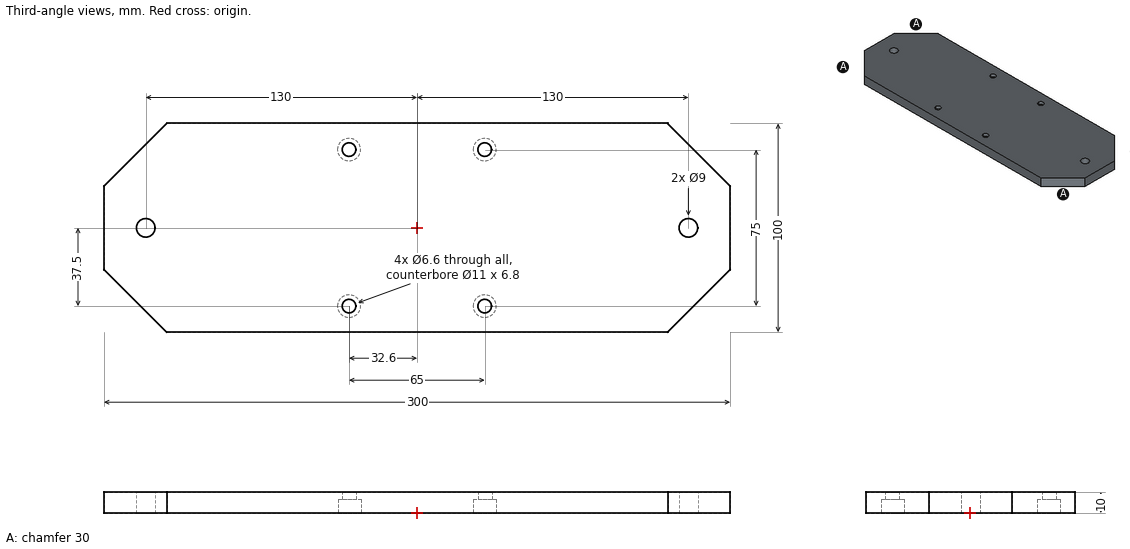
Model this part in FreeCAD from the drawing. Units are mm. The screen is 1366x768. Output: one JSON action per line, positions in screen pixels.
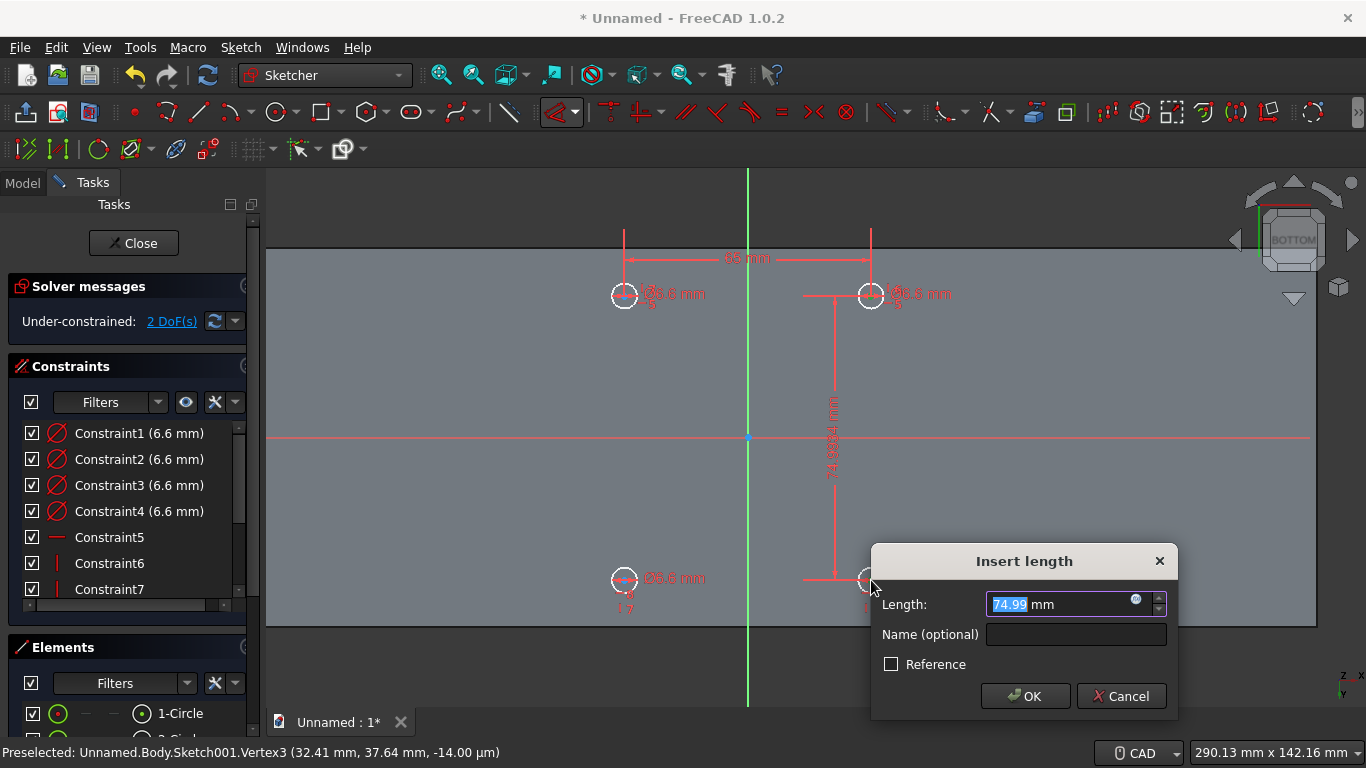
{"action": "type", "text": "75"}
{"action": "key", "text": "Return"}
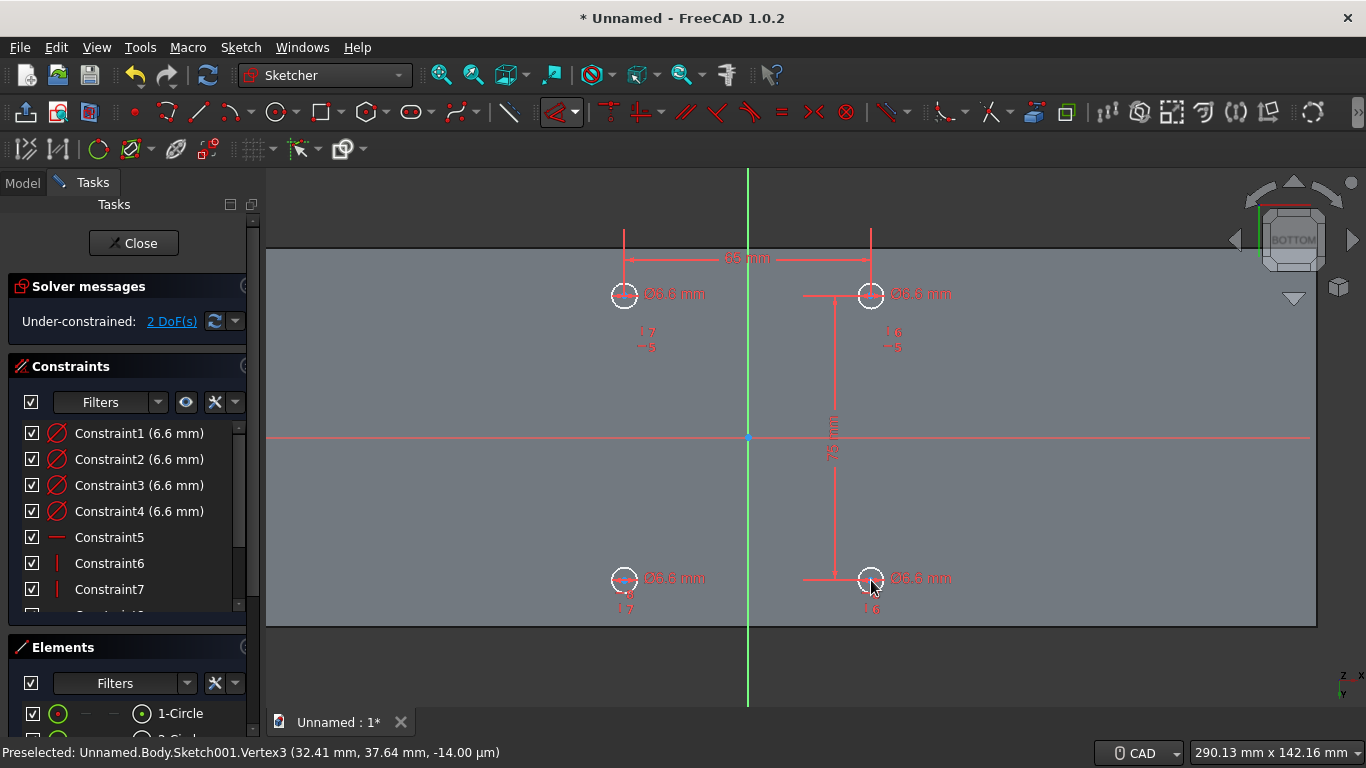
{"action": "left_click", "coordinate": [625, 296]}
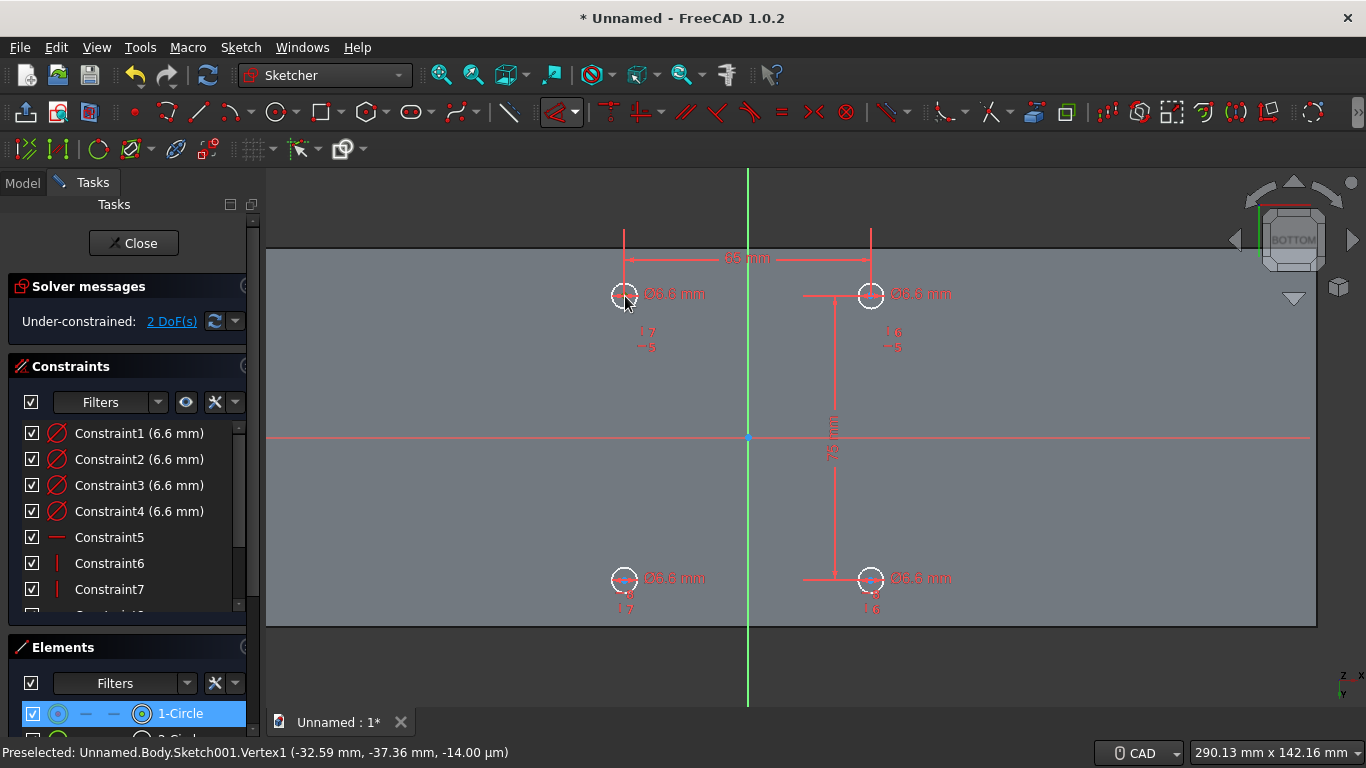
{"action": "key", "text": "l"}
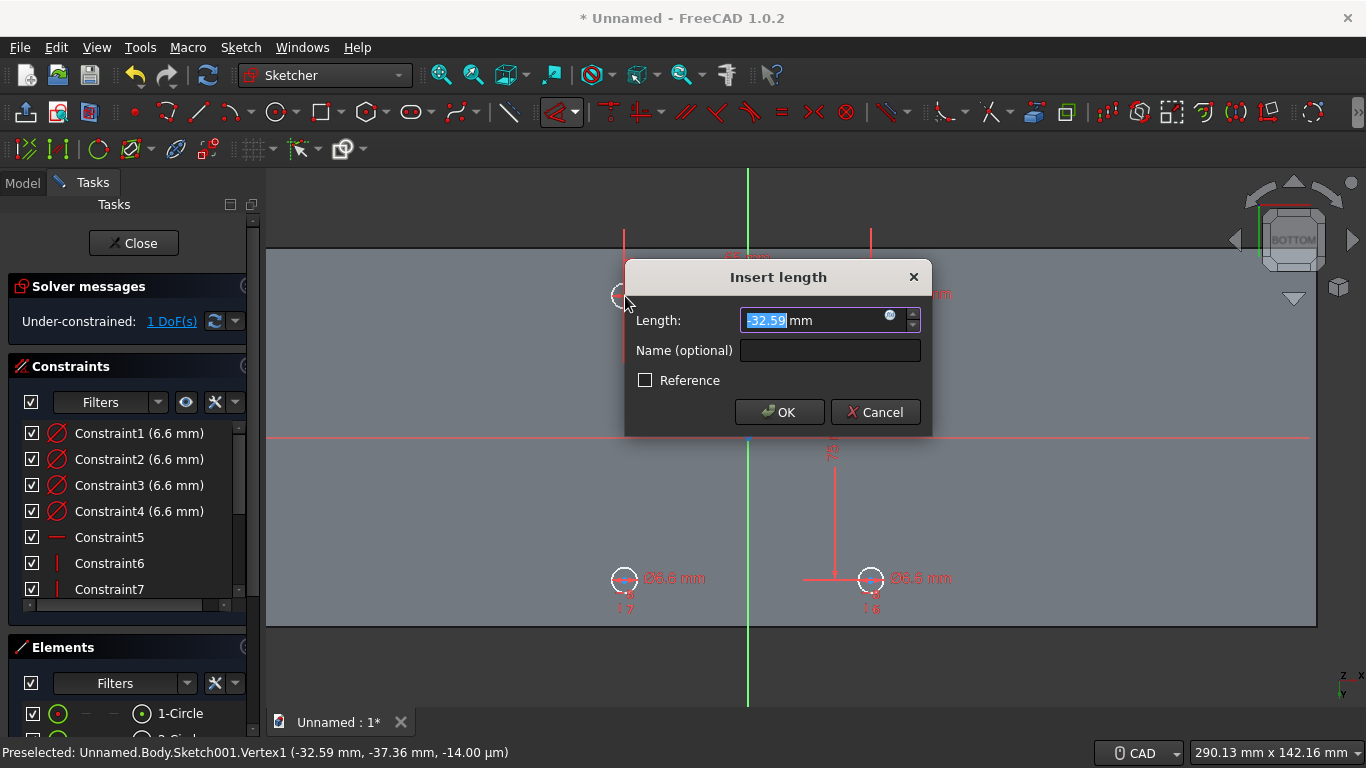
{"action": "type", "text": "-32.6"}
{"action": "key", "text": "Return"}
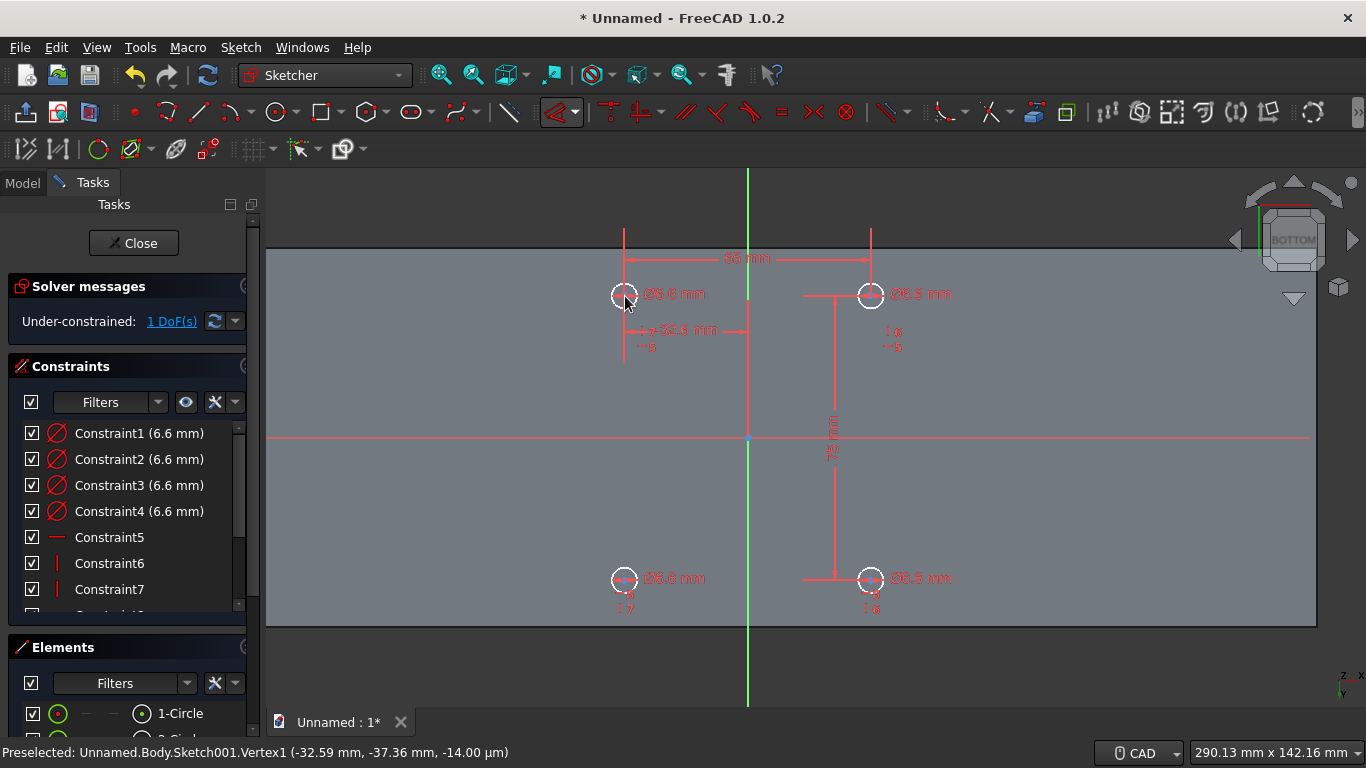
{"action": "left_click", "coordinate": [624, 296]}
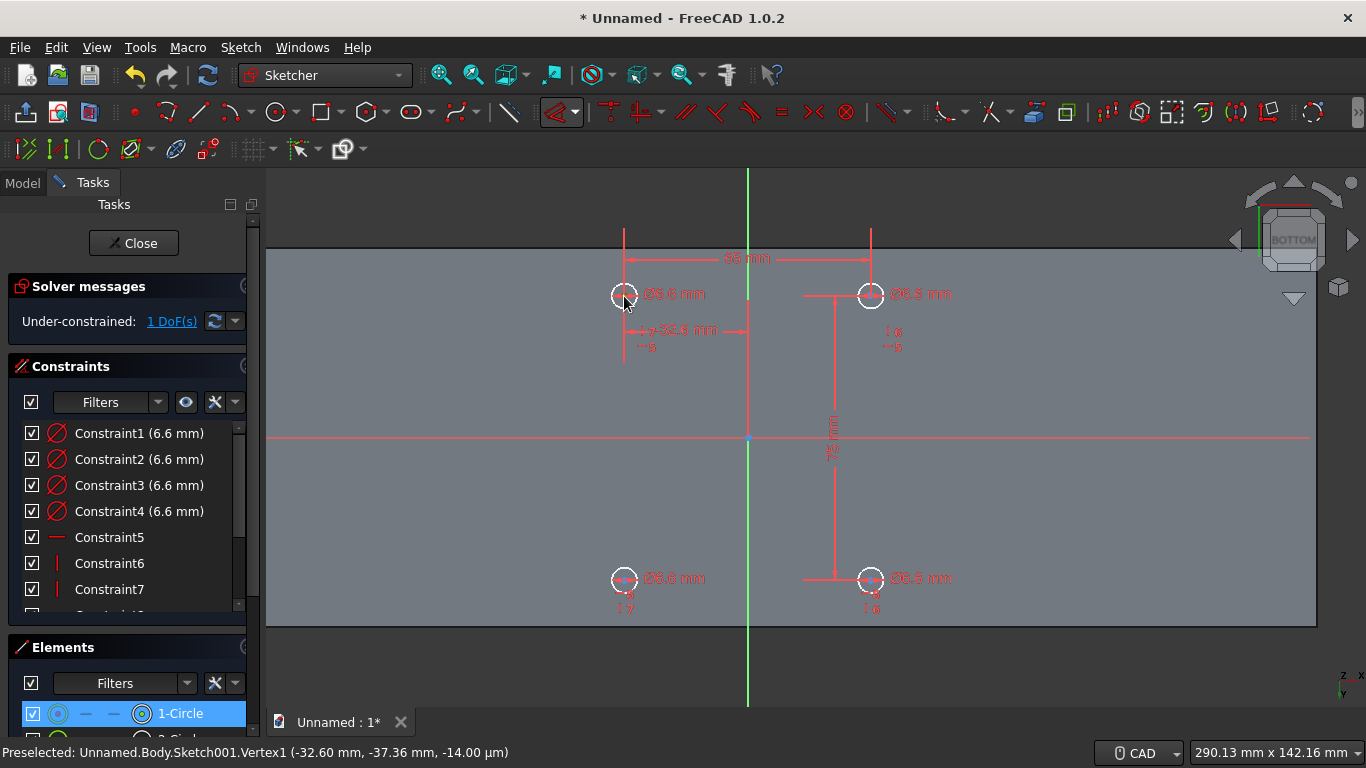
{"action": "key", "text": "i"}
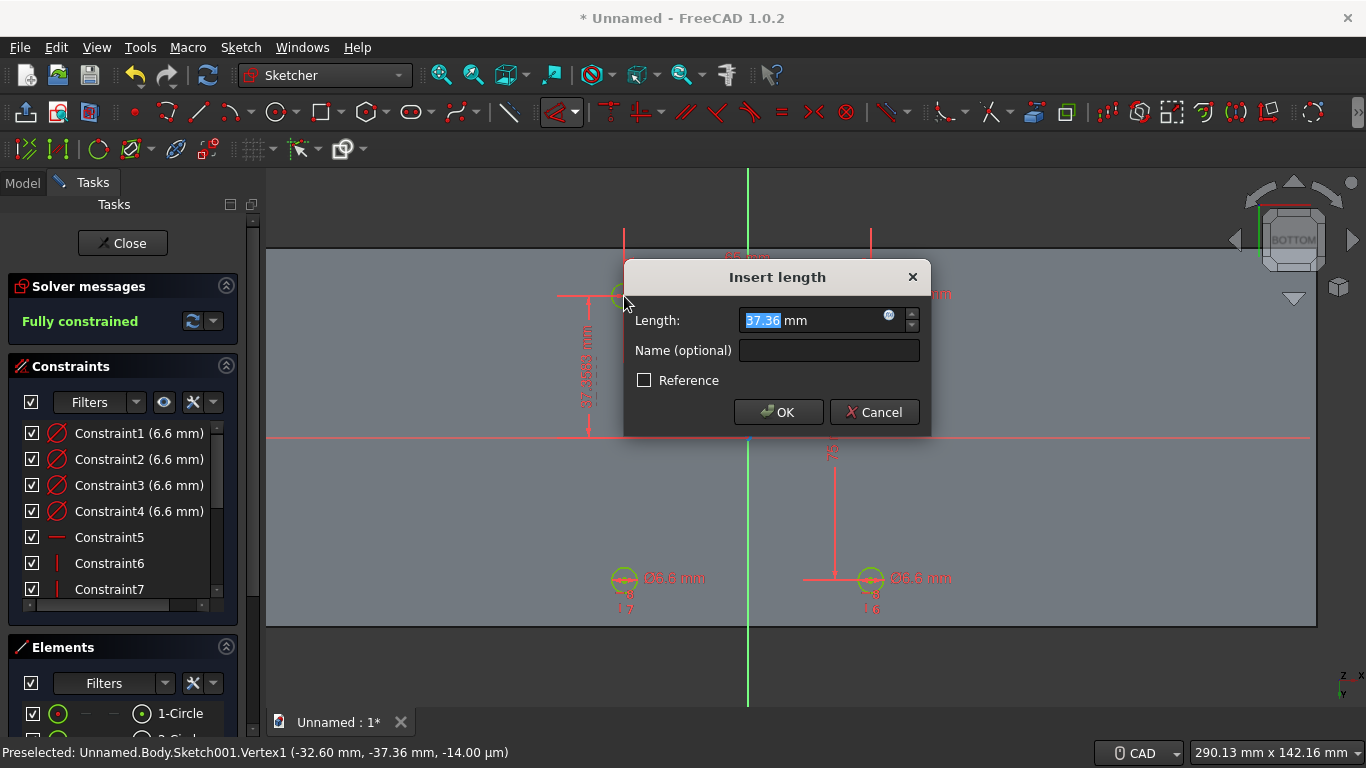
{"action": "type", "text": "37.5"}
{"action": "key", "text": "Return"}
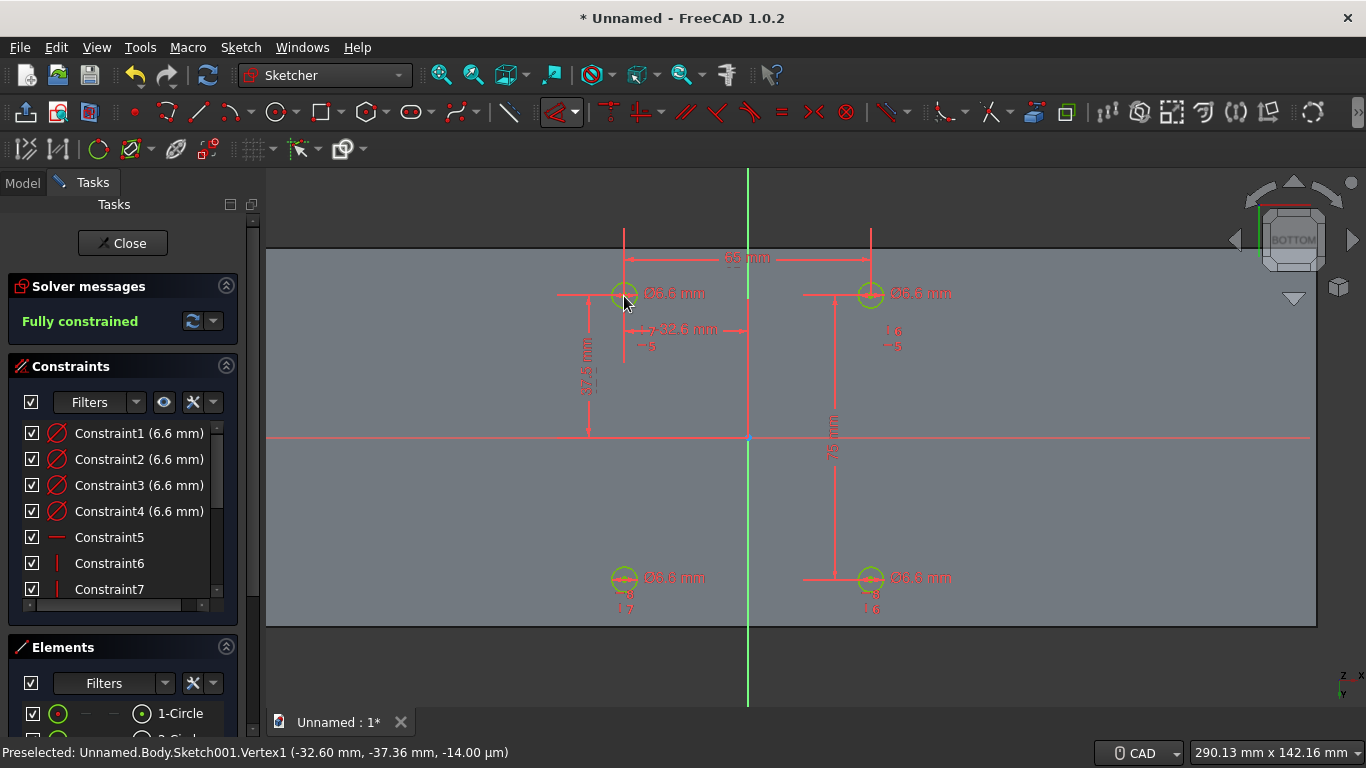
{"action": "left_click", "coordinate": [123, 243]}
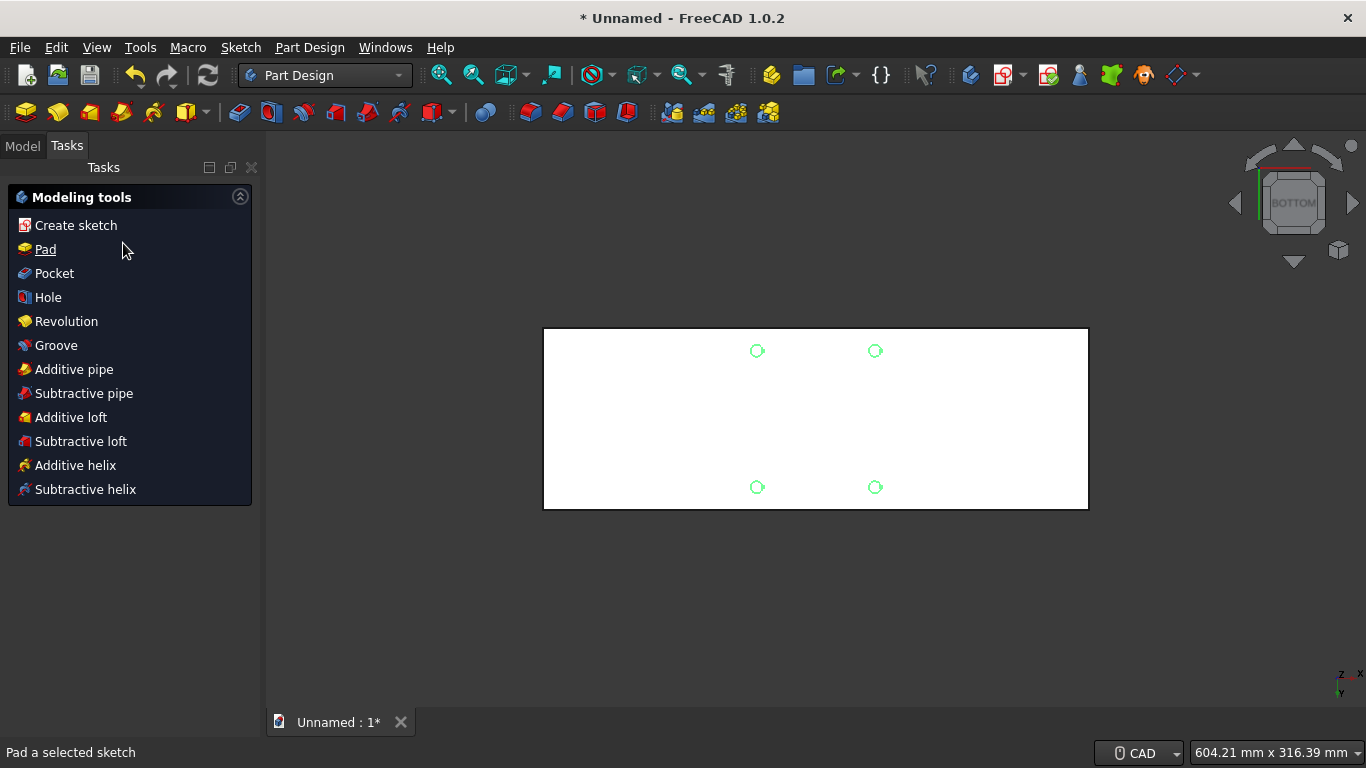
{"action": "left_click", "coordinate": [272, 112]}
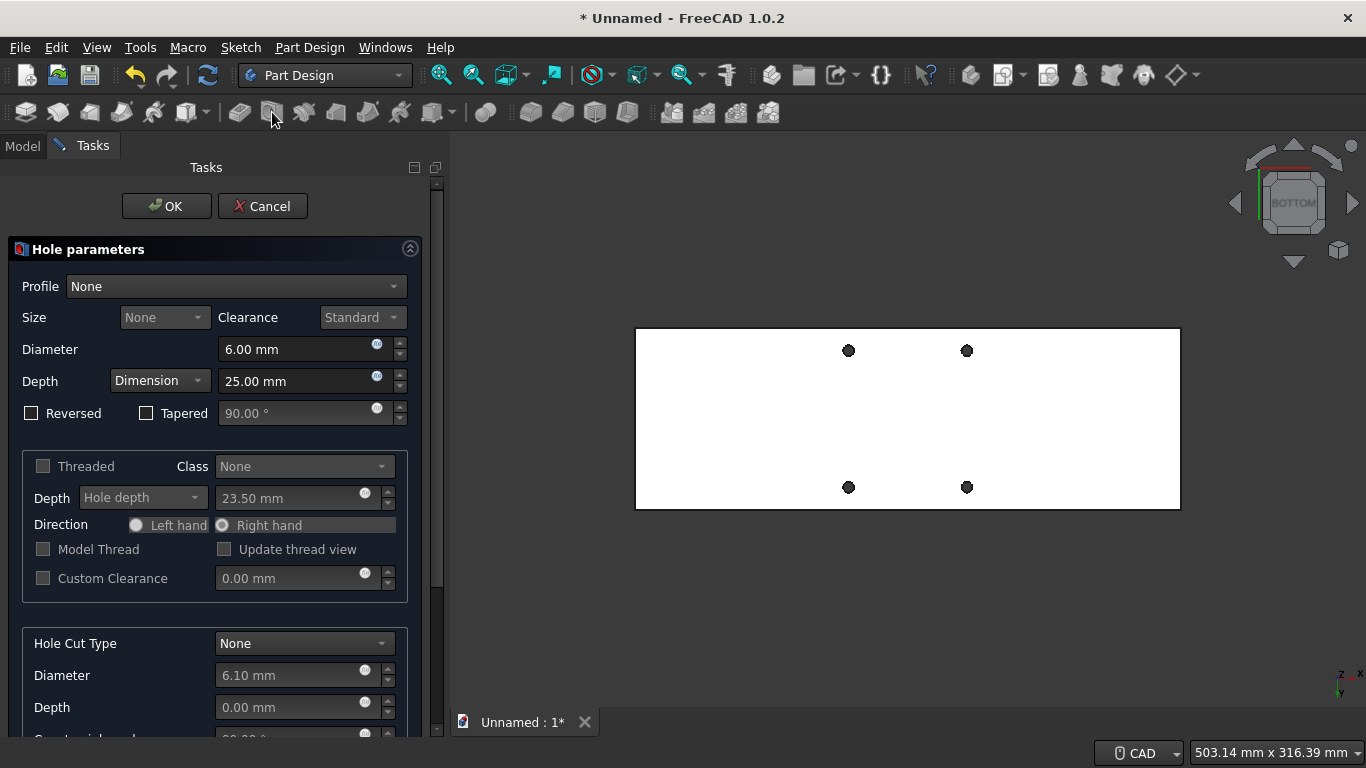
{"action": "triple_click", "coordinate": [305, 349]}